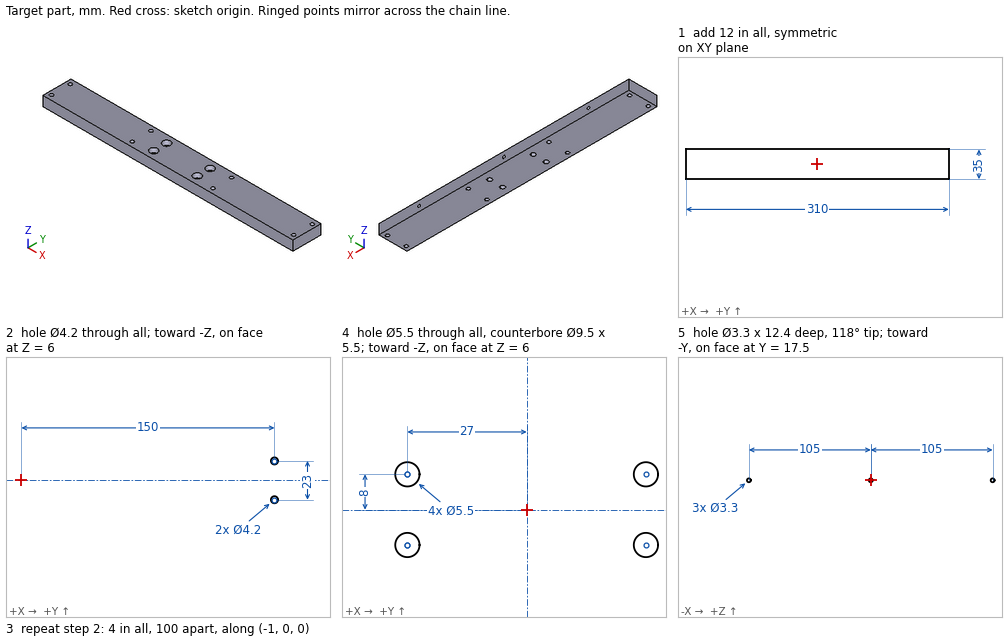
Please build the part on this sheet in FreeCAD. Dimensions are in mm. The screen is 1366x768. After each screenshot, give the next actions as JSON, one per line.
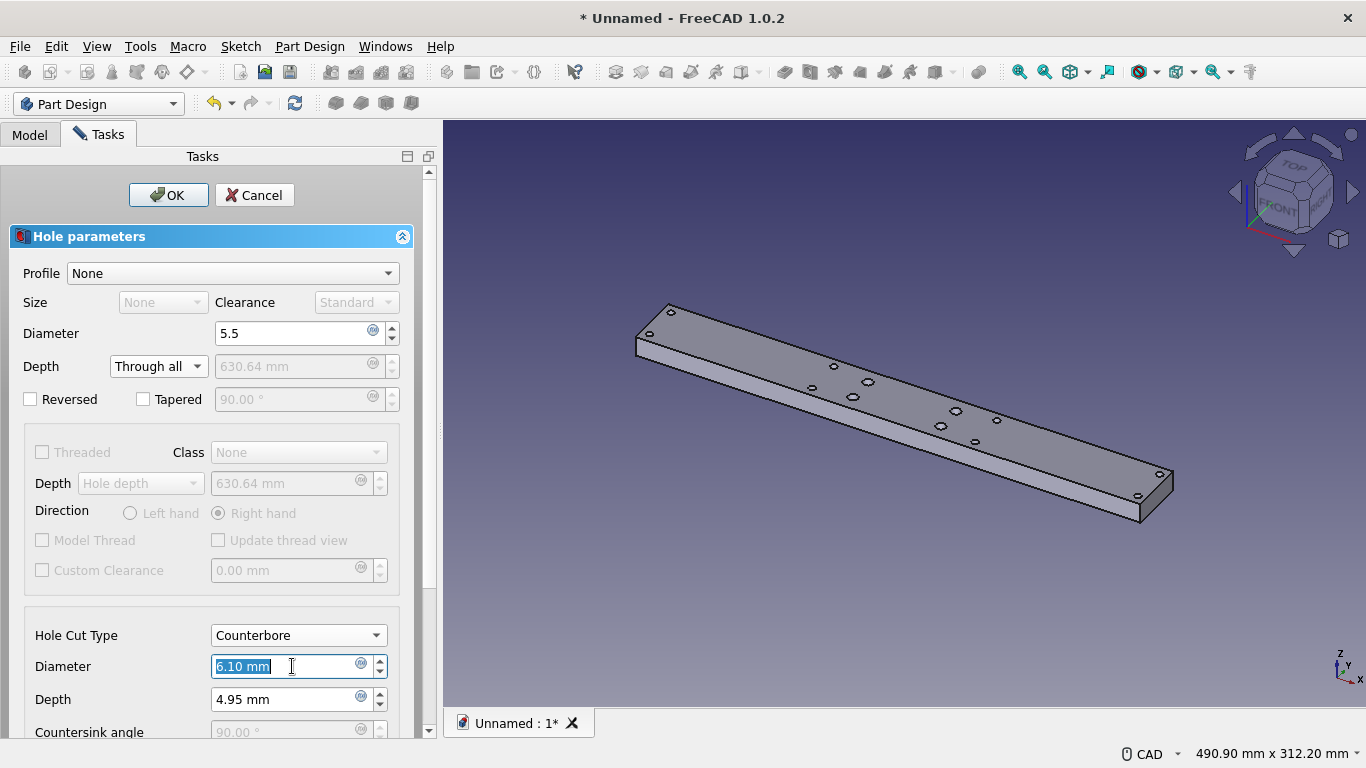
{"action": "type", "text": "9.5"}
{"action": "key", "text": "Tab"}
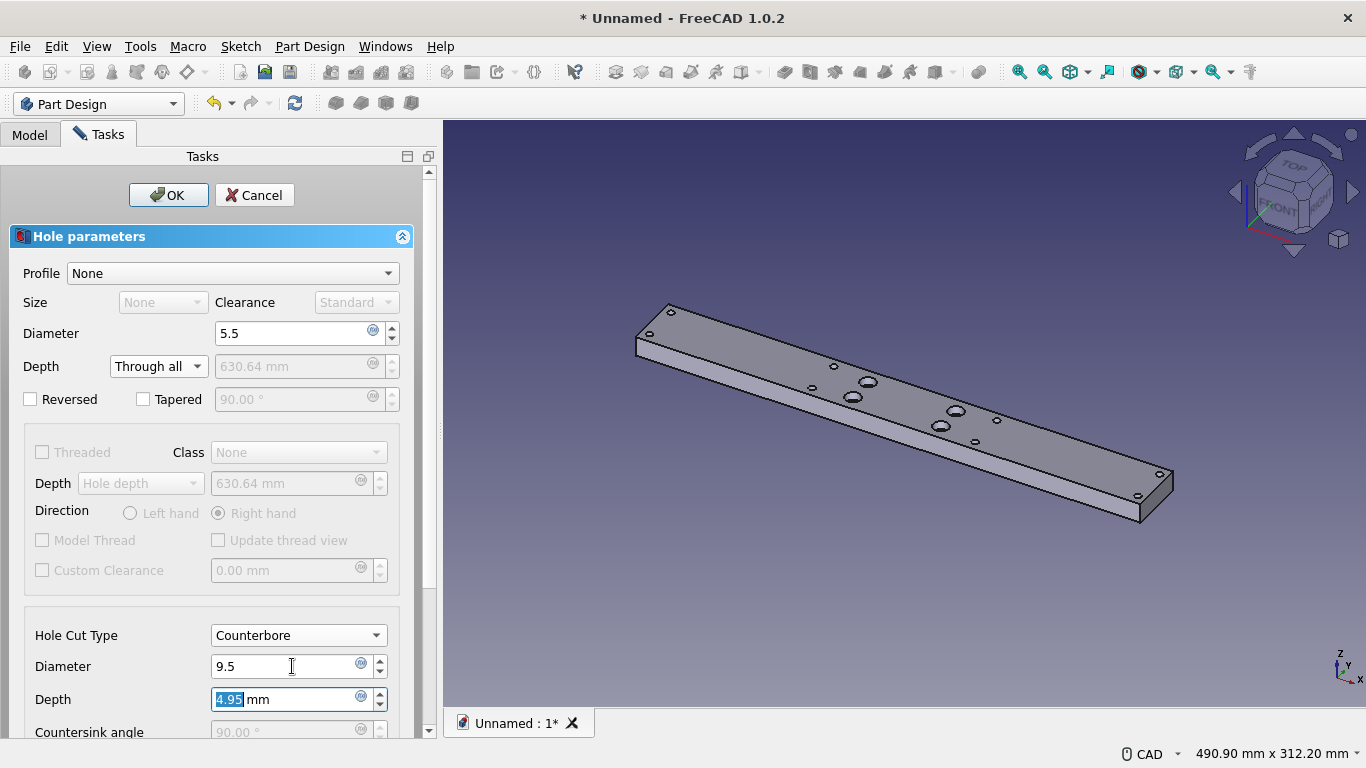
{"action": "type", "text": "5.5"}
{"action": "key", "text": "Tab"}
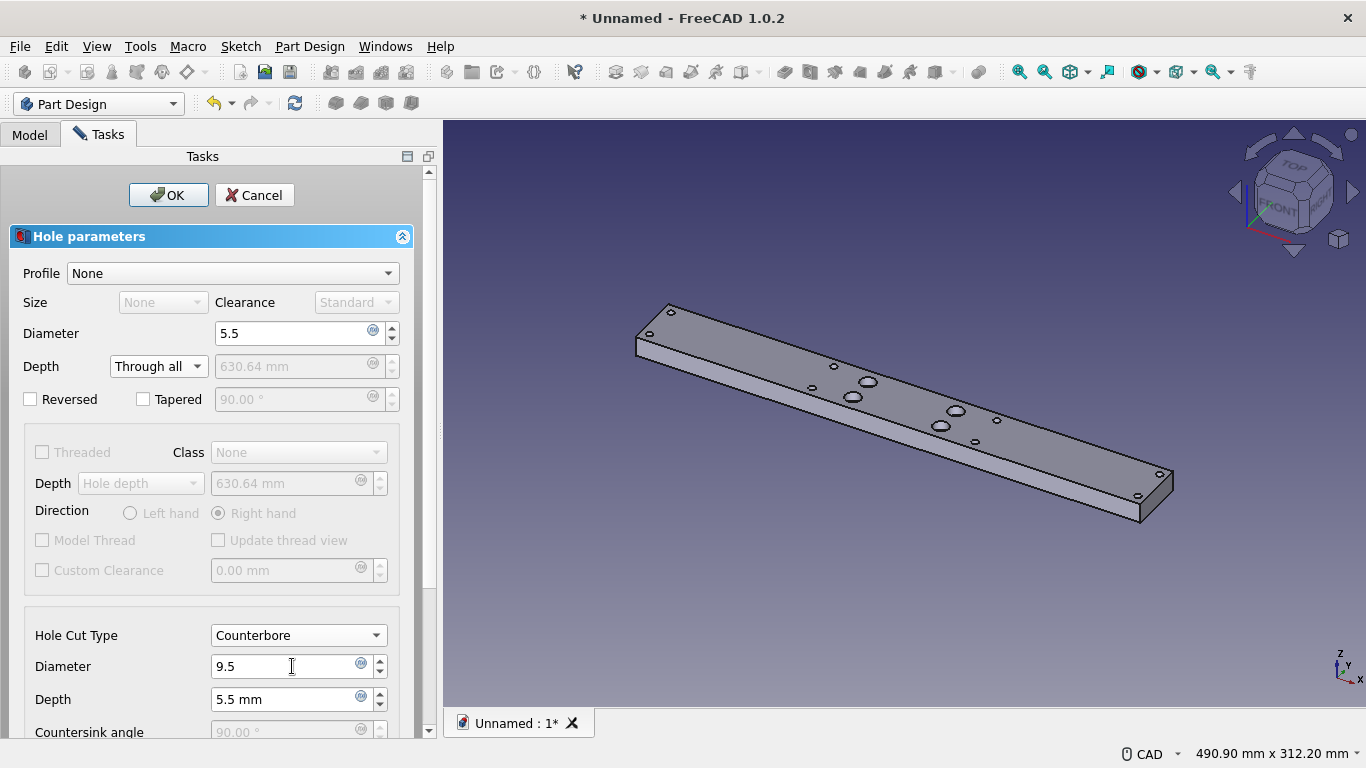
{"action": "left_click", "coordinate": [169, 195]}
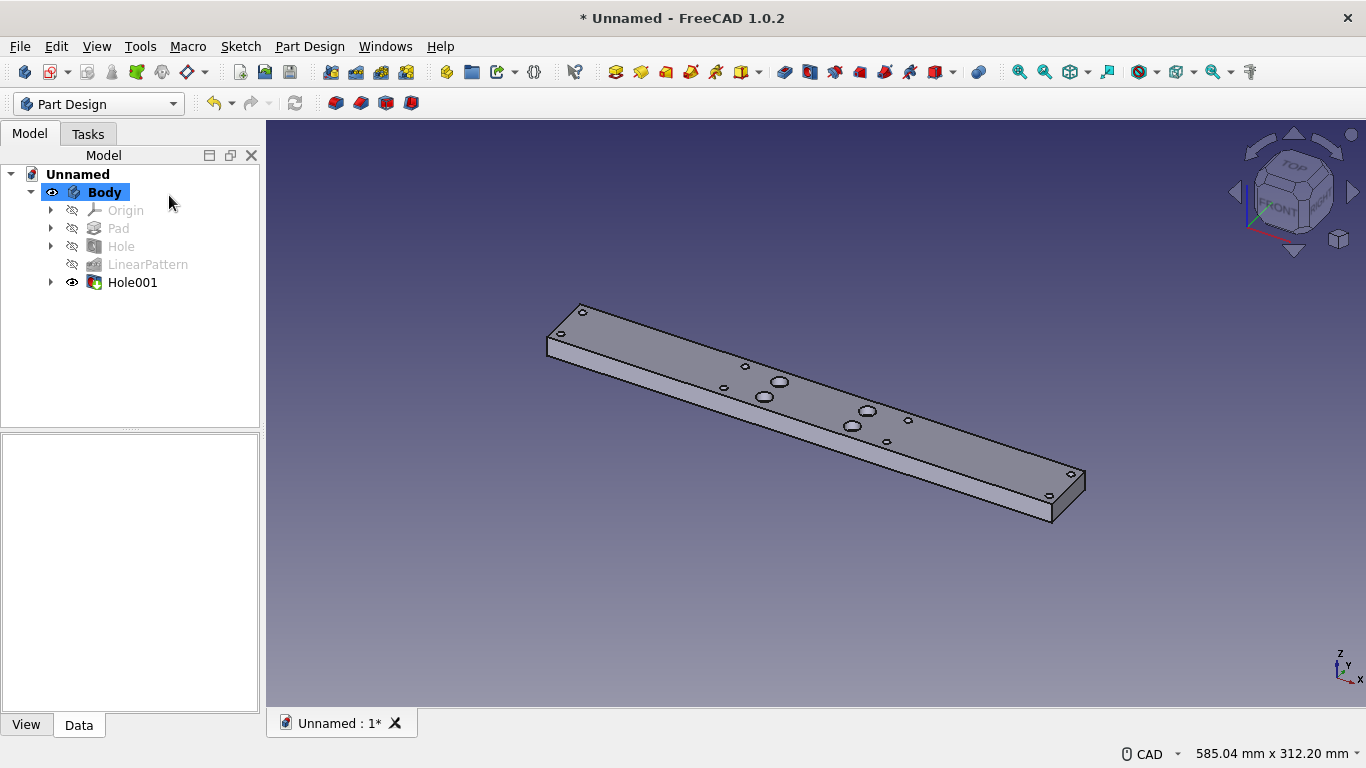
{"action": "key", "text": "4"}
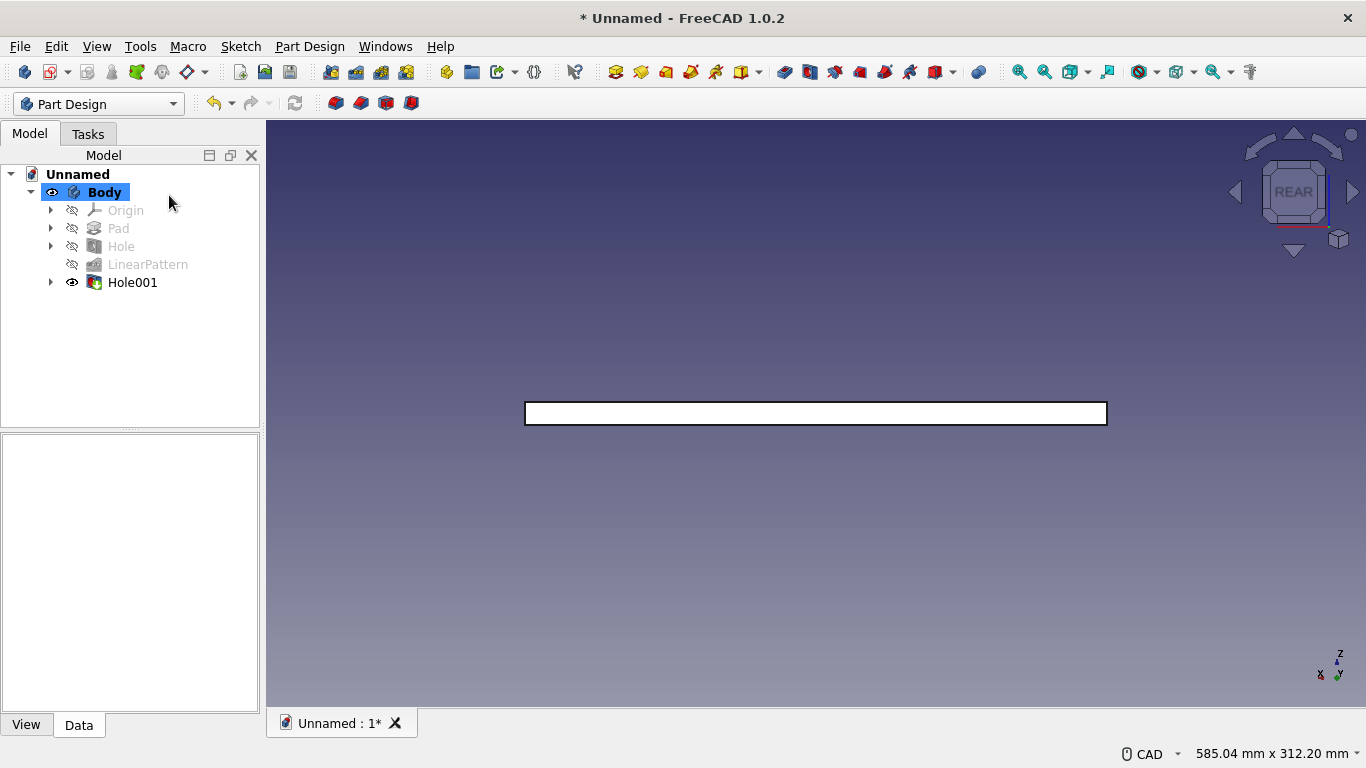
{"action": "left_click", "coordinate": [566, 413]}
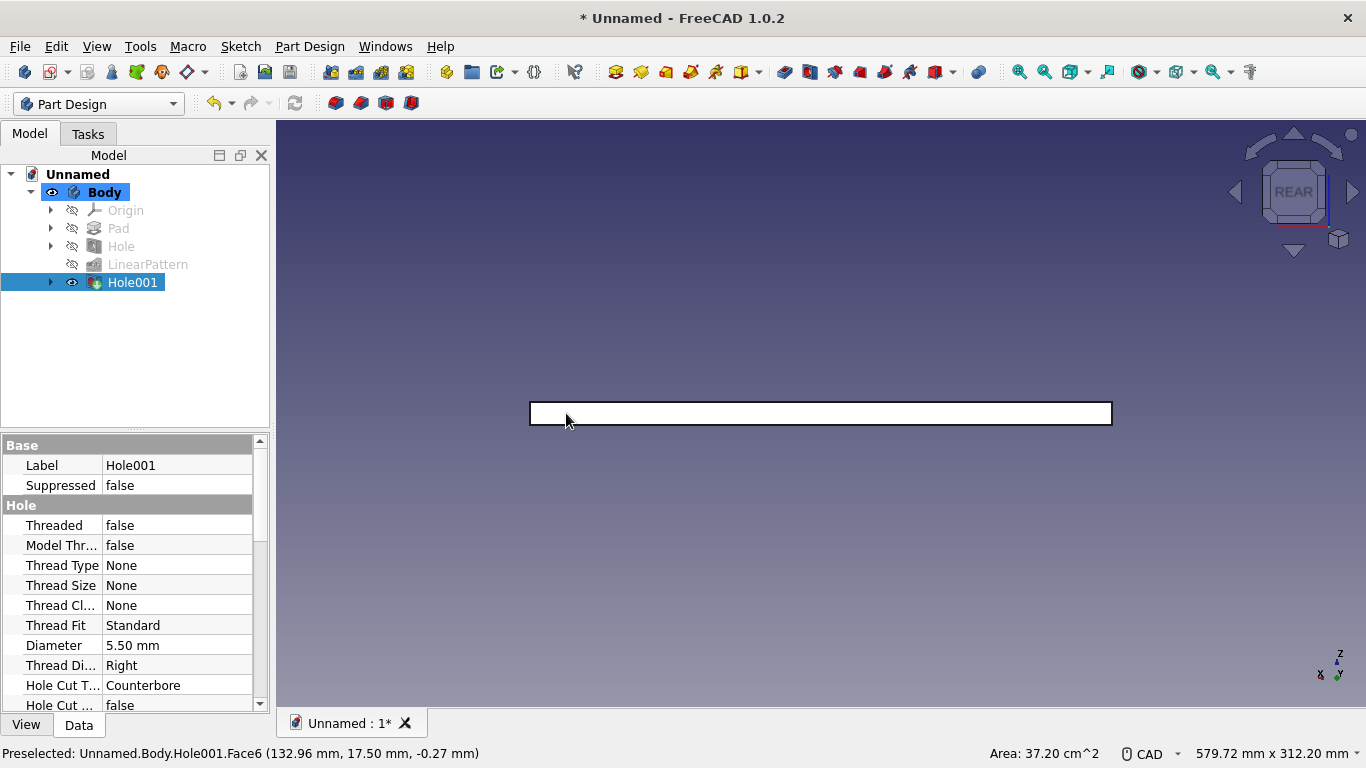
{"action": "left_click", "coordinate": [50, 72]}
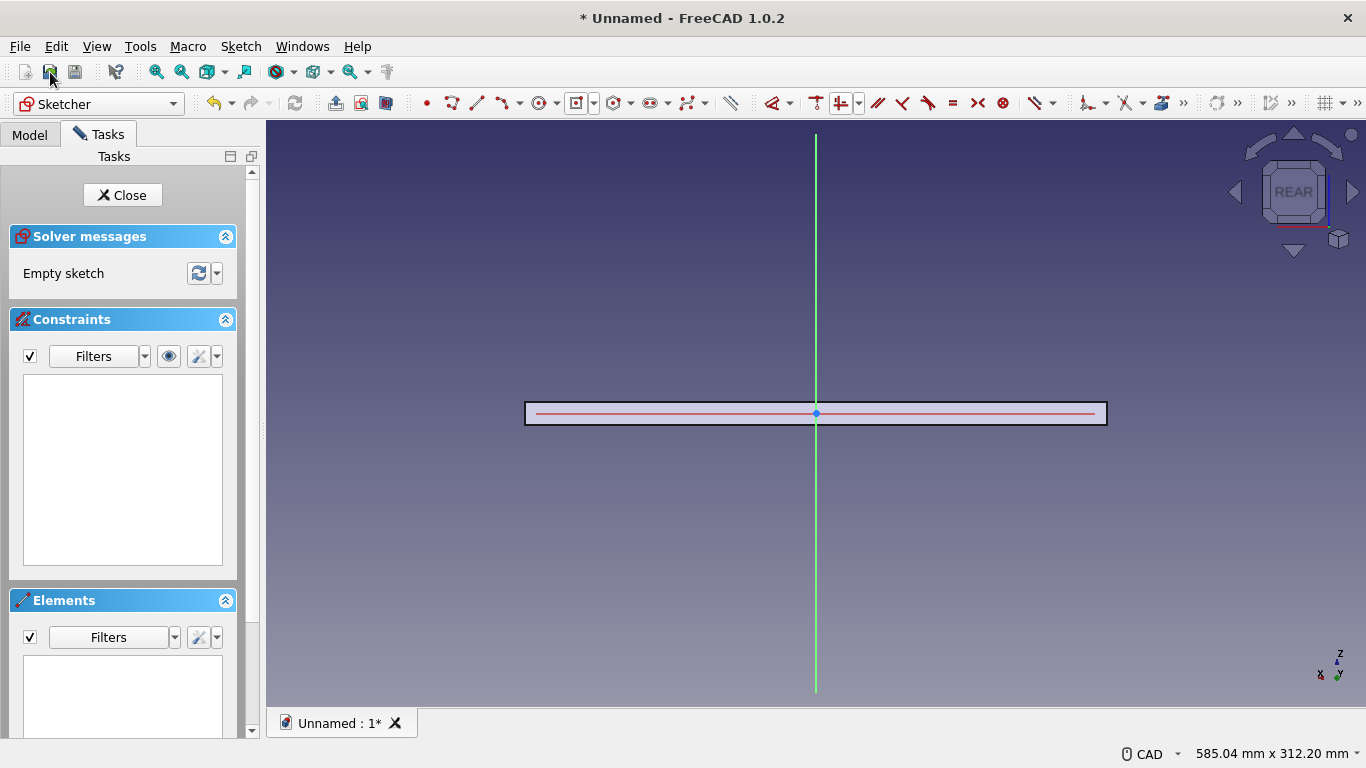
{"action": "scroll", "coordinate": [955, 414], "scroll_direction": "up", "scroll_amount": 2}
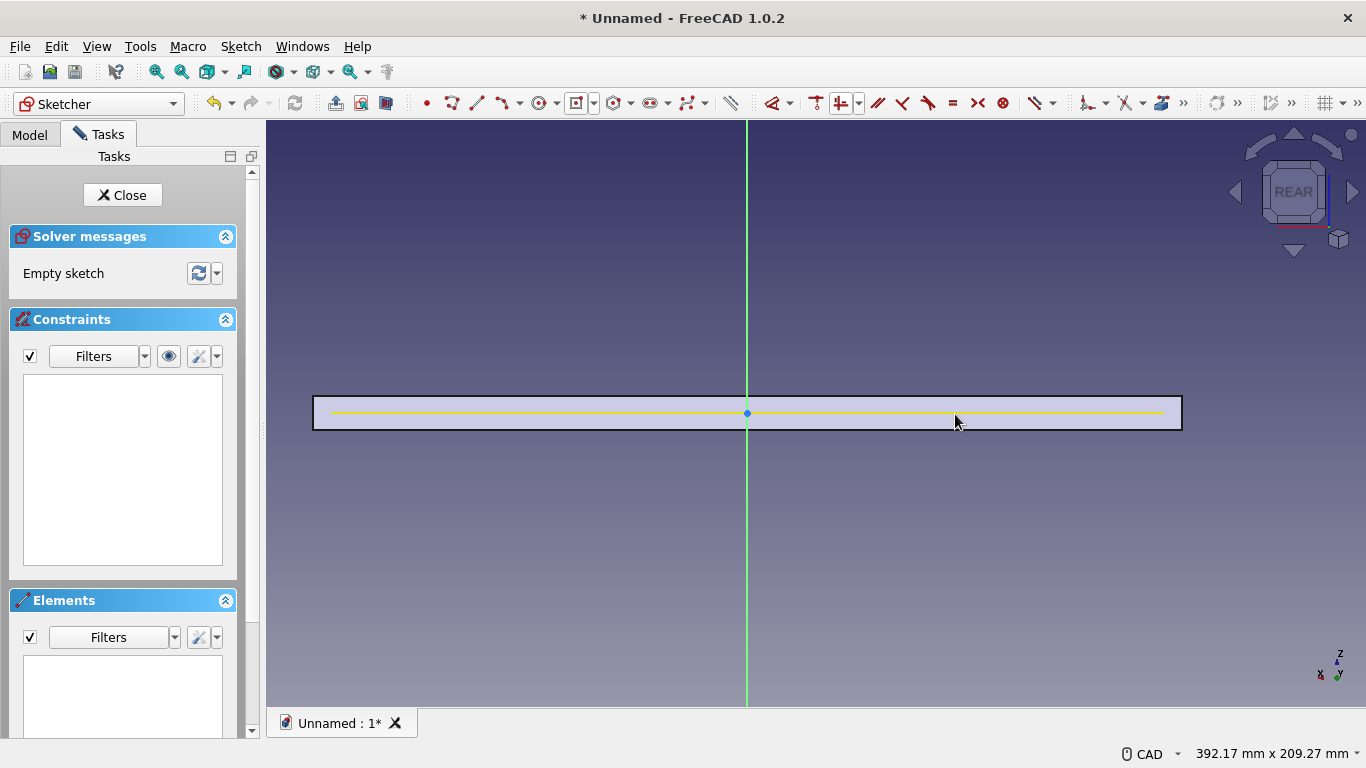
{"action": "left_click", "coordinate": [538, 104]}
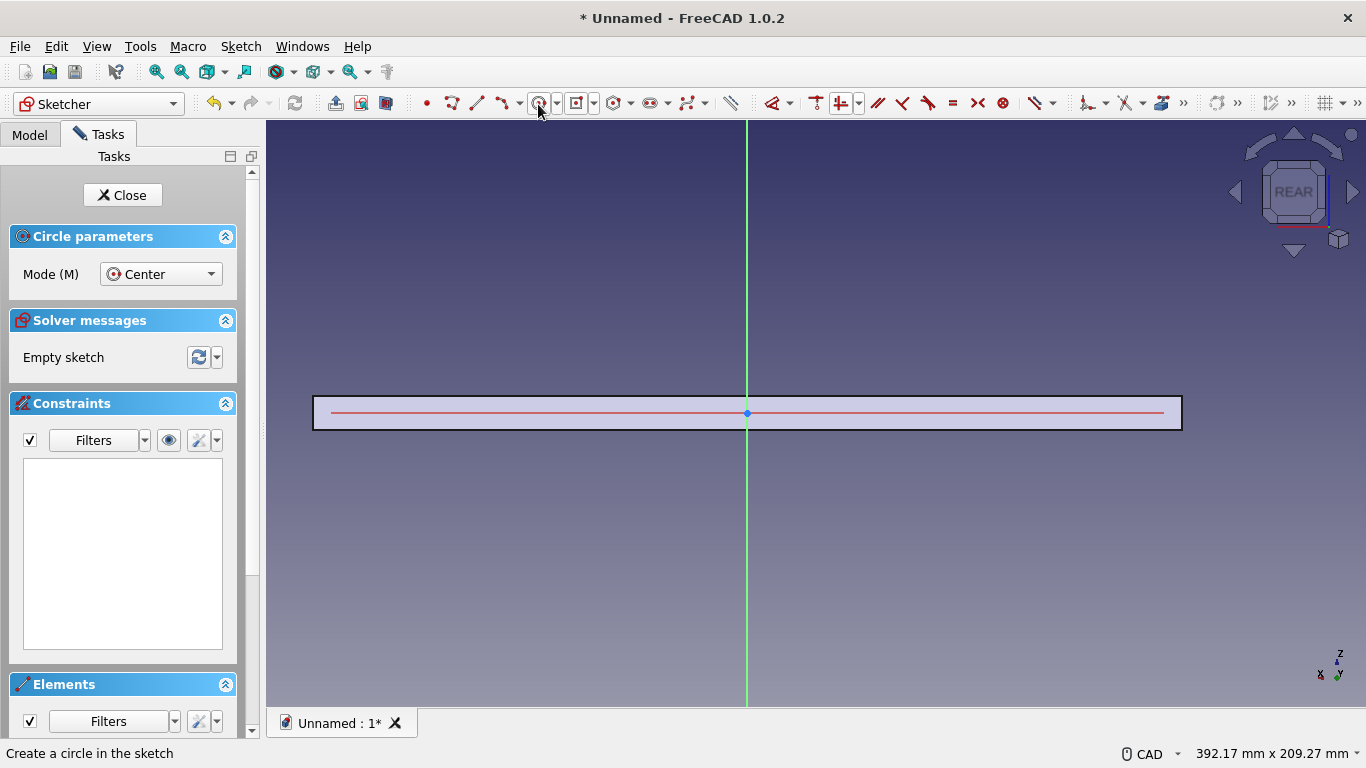
{"action": "scroll", "coordinate": [453, 413], "scroll_direction": "up", "scroll_amount": 8}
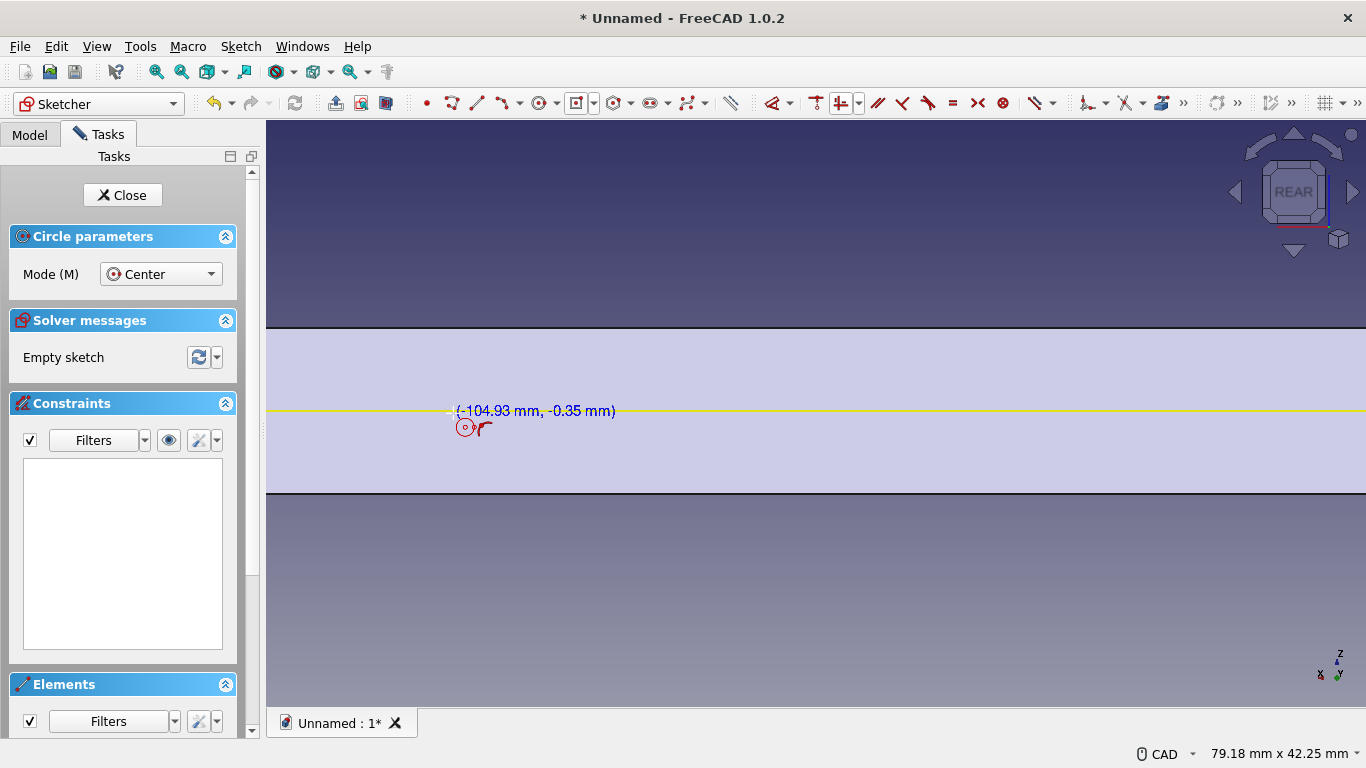
{"action": "scroll", "coordinate": [453, 414], "scroll_direction": "down", "scroll_amount": 8}